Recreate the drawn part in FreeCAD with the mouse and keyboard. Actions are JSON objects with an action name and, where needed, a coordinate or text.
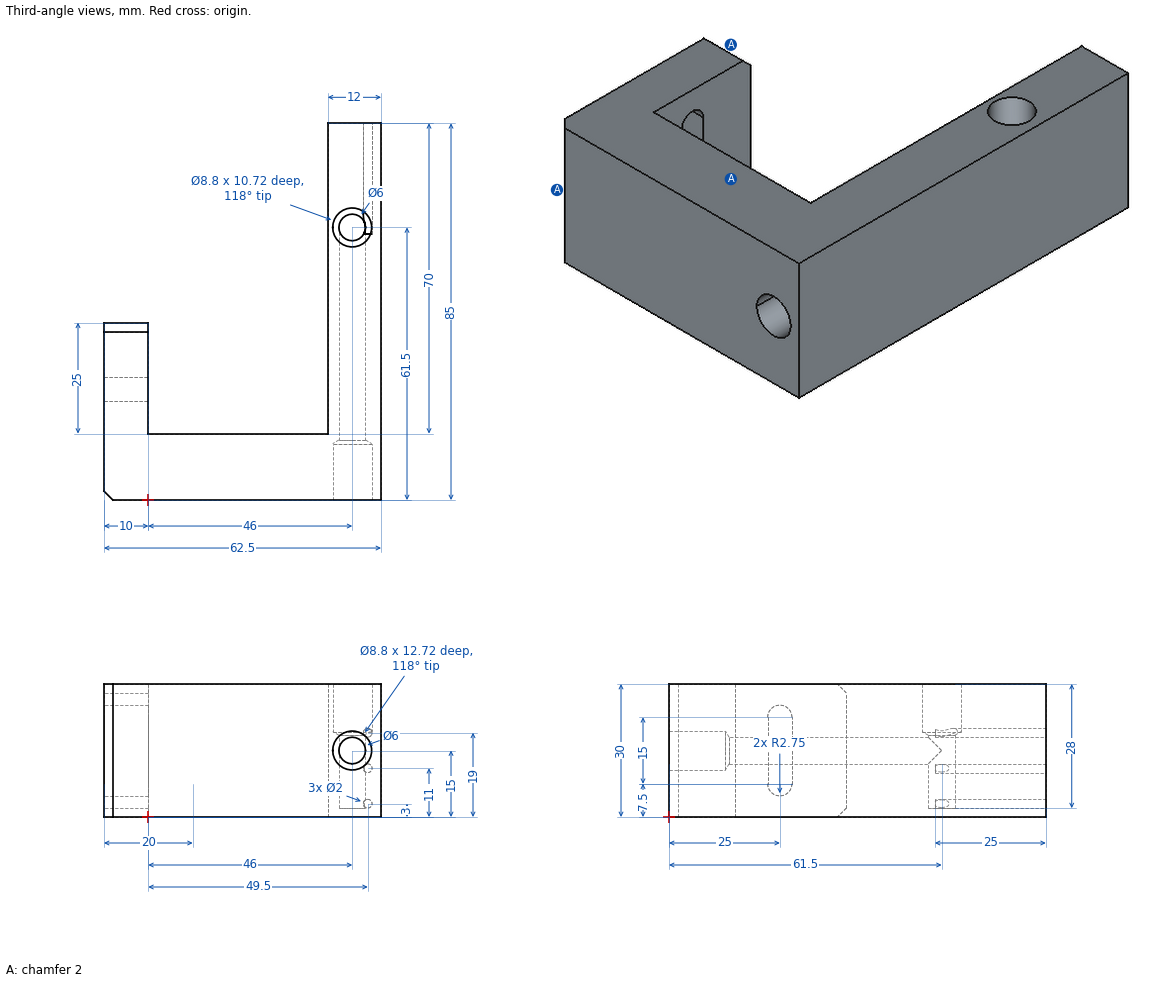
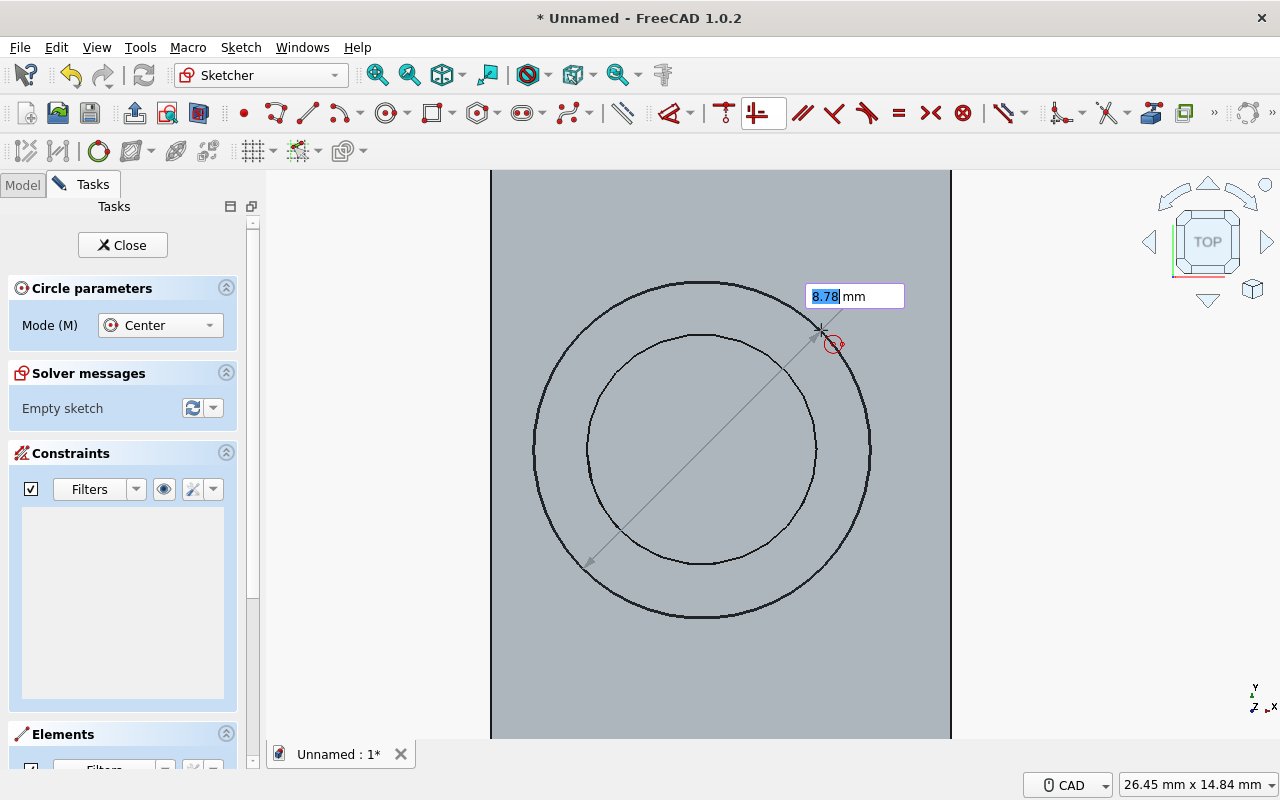
{"action": "type", "text": "8.8"}
{"action": "key", "text": "Return"}
{"action": "key", "text": "Escape"}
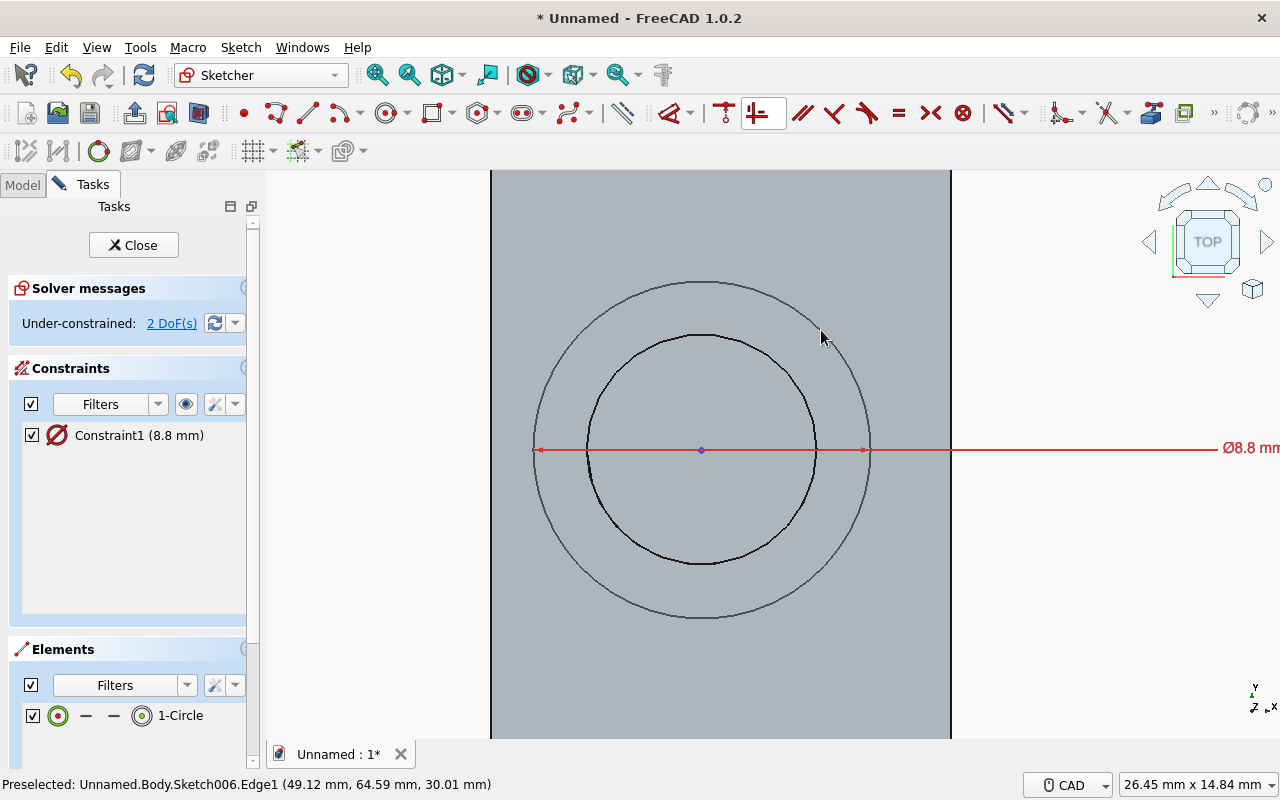
{"action": "key", "text": "d"}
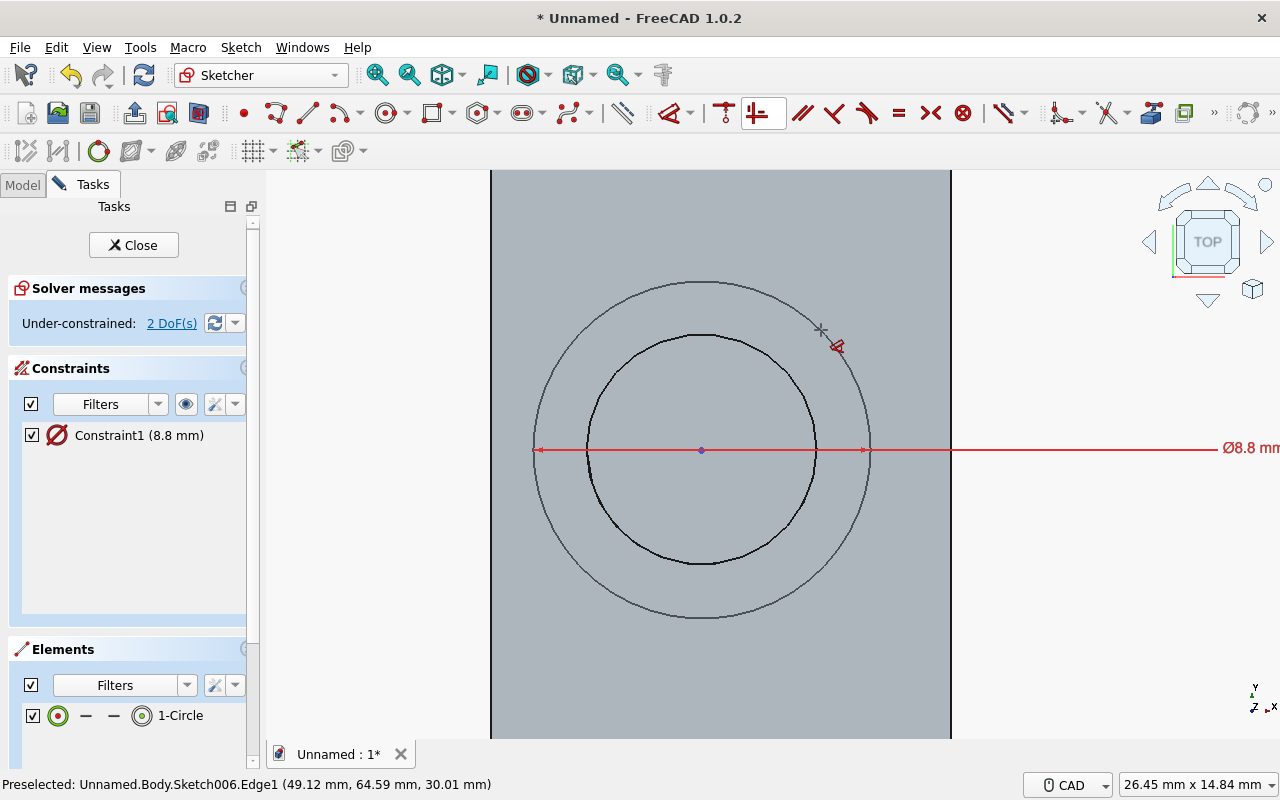
{"action": "left_click", "coordinate": [702, 450]}
{"action": "left_click", "coordinate": [498, 416]}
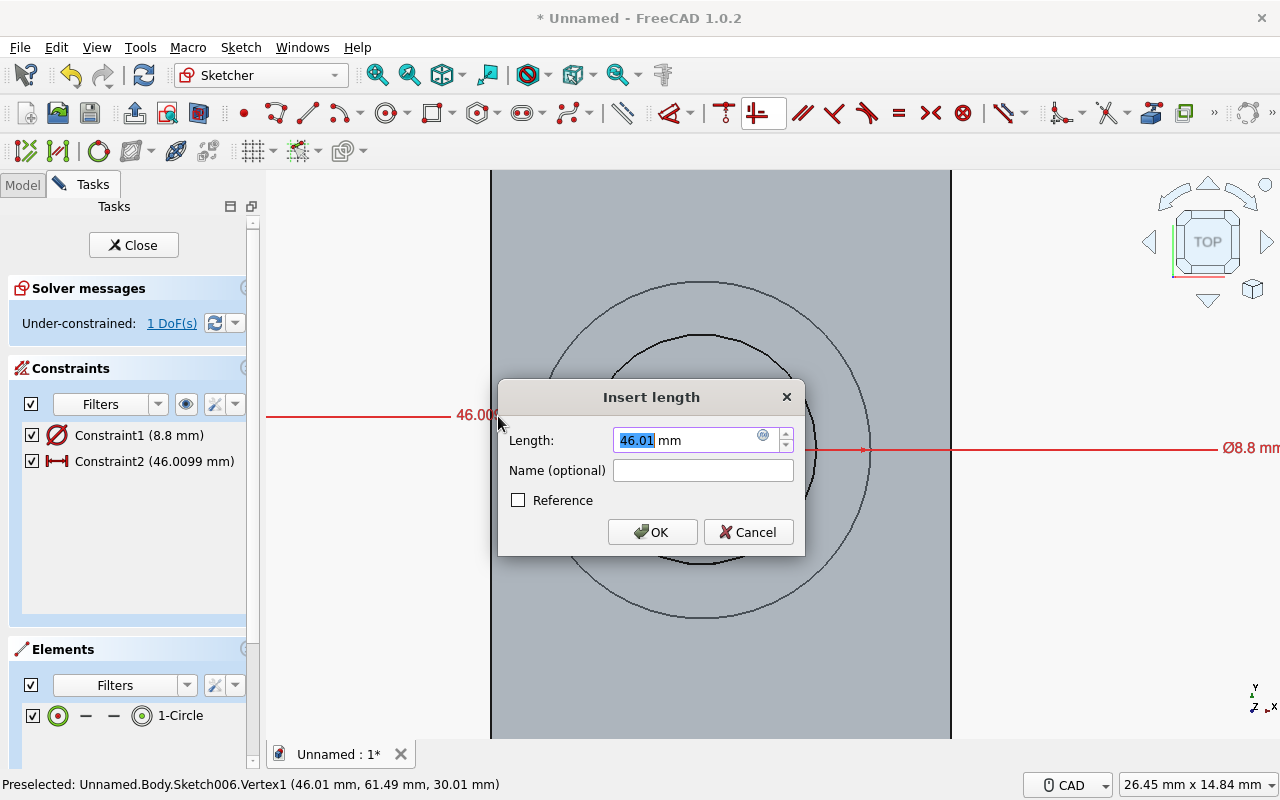
{"action": "type", "text": "46"}
{"action": "key", "text": "Return"}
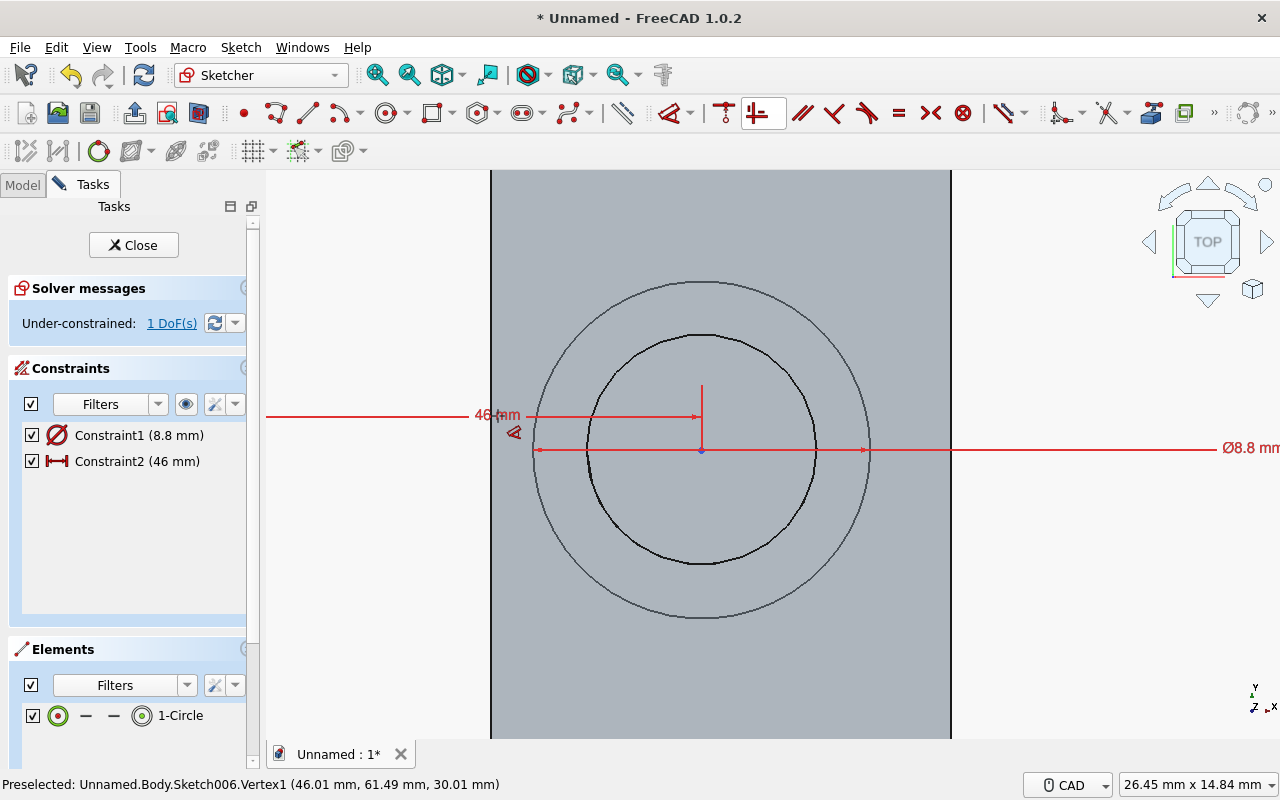
{"action": "left_click", "coordinate": [702, 450]}
{"action": "left_click", "coordinate": [736, 581]}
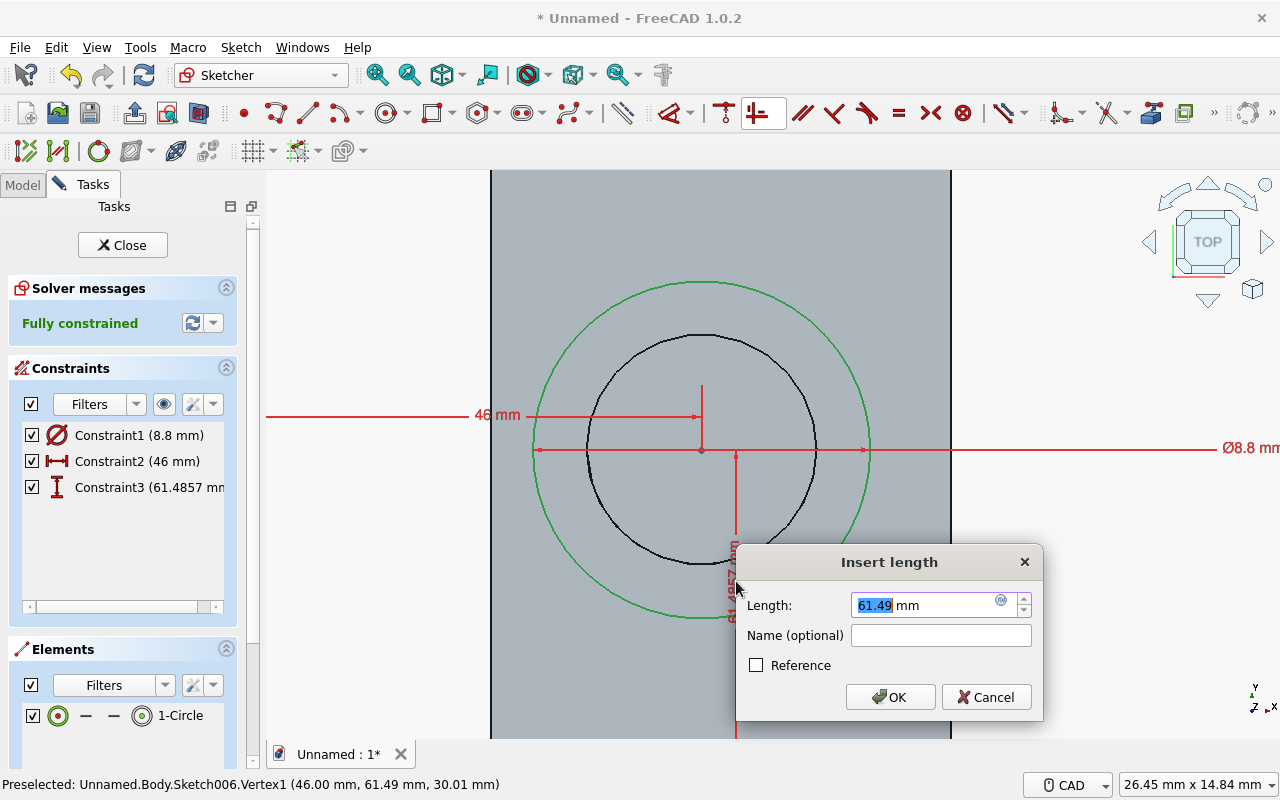
{"action": "type", "text": "61.5"}
{"action": "key", "text": "Return"}
{"action": "key", "text": "Escape"}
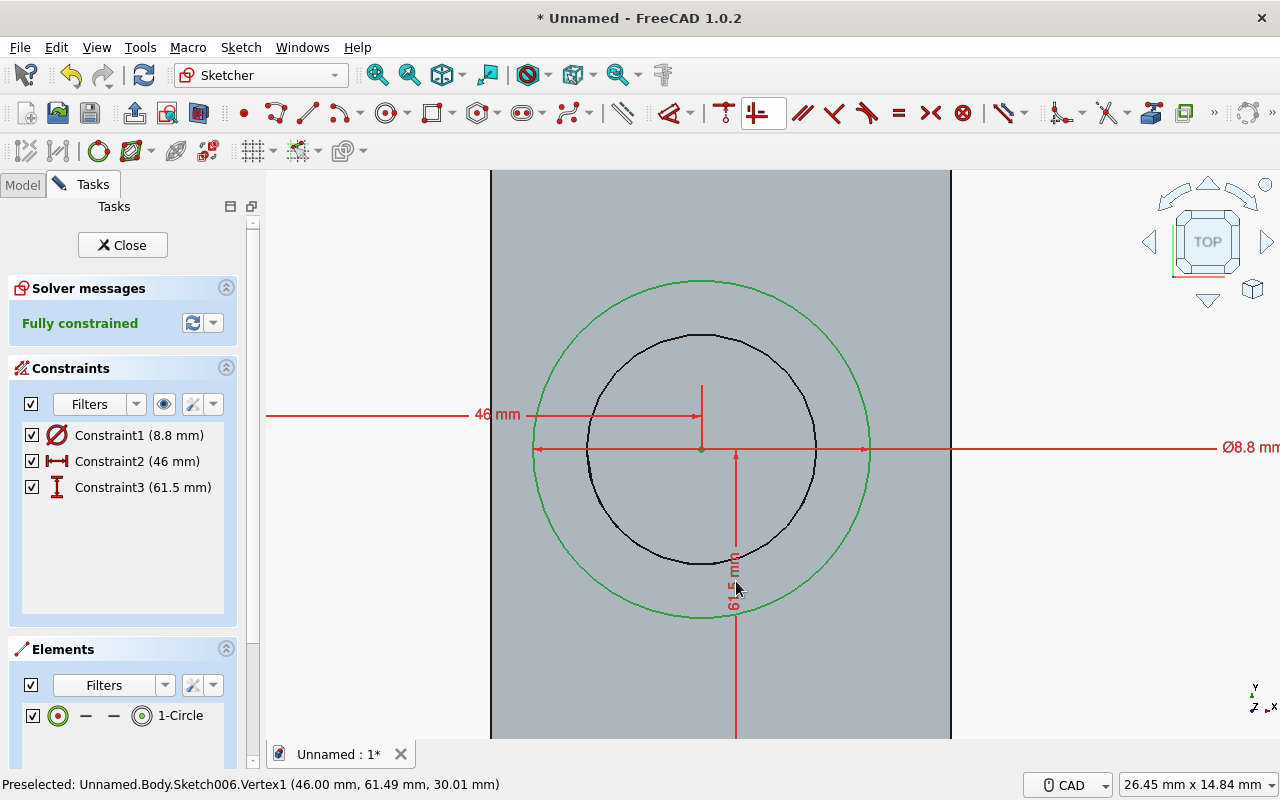
{"action": "left_click", "coordinate": [123, 245]}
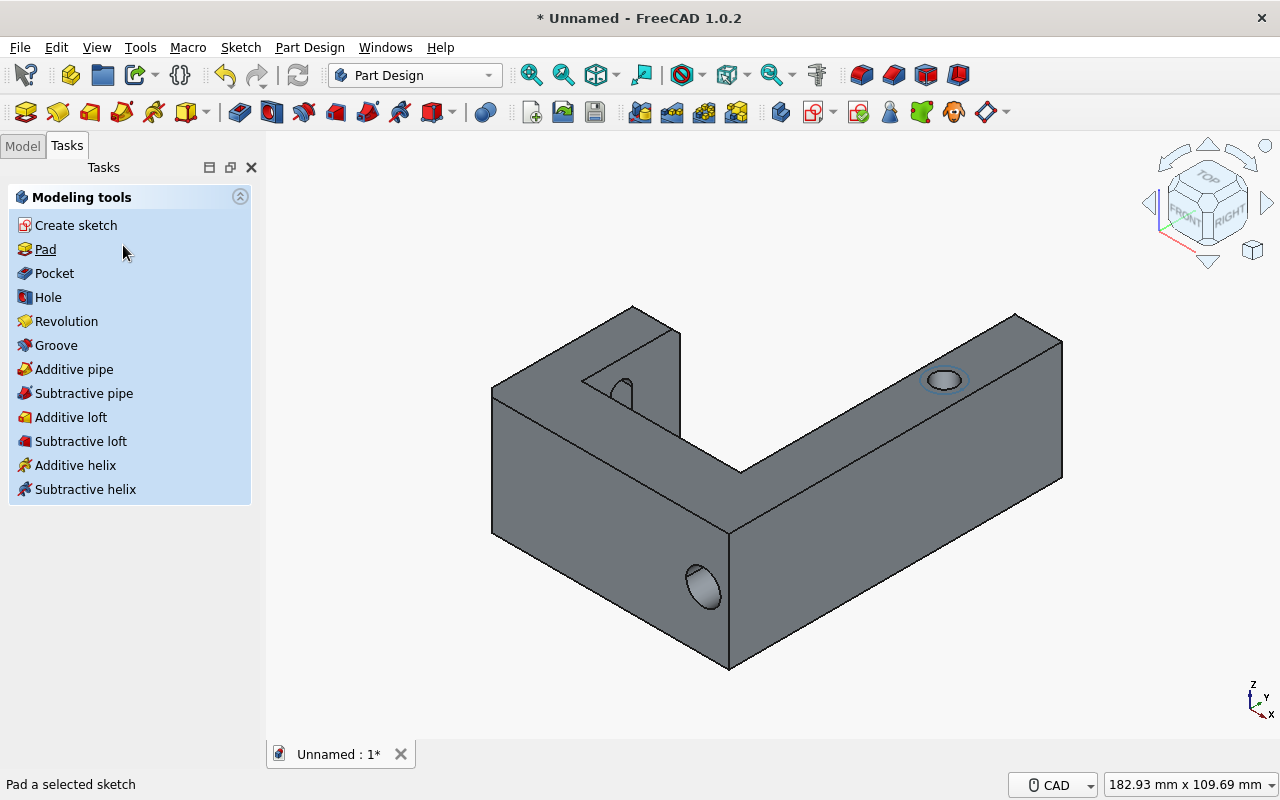
{"action": "left_click", "coordinate": [272, 112]}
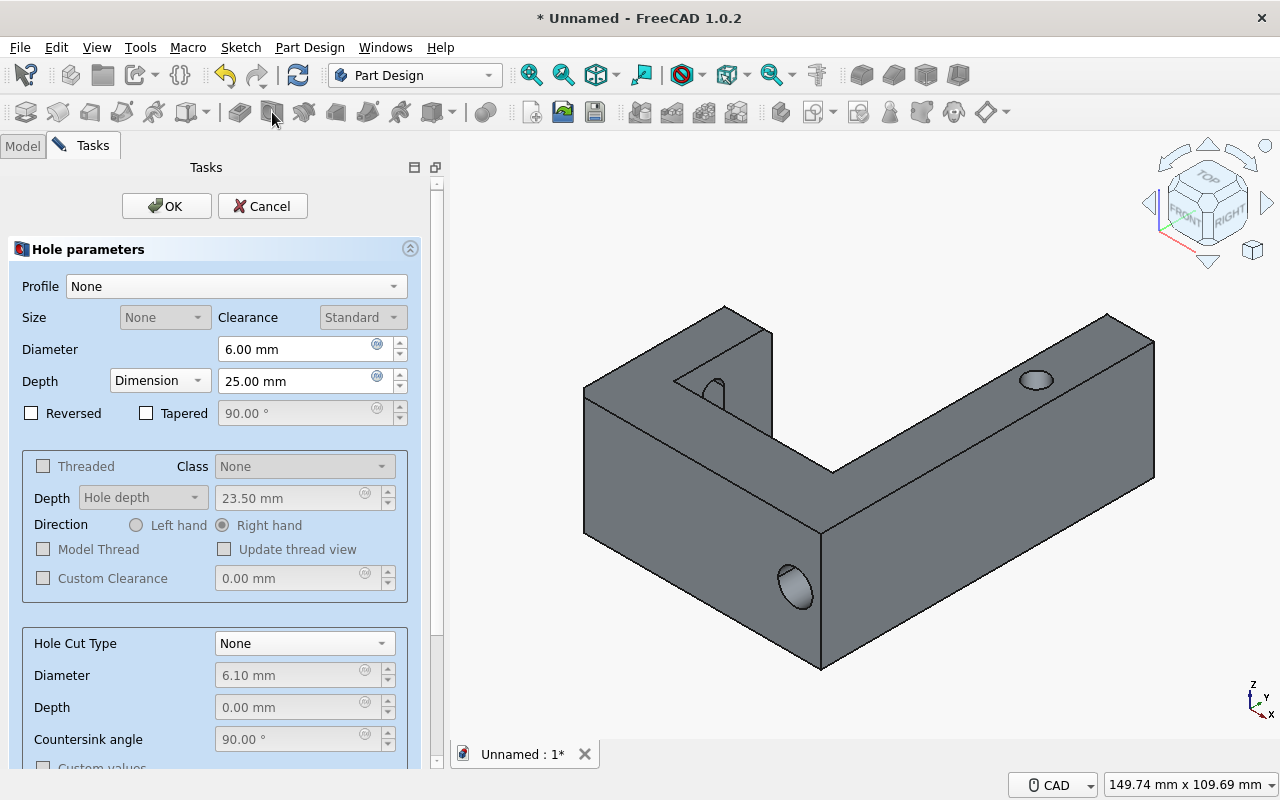
{"action": "triple_click", "coordinate": [305, 349]}